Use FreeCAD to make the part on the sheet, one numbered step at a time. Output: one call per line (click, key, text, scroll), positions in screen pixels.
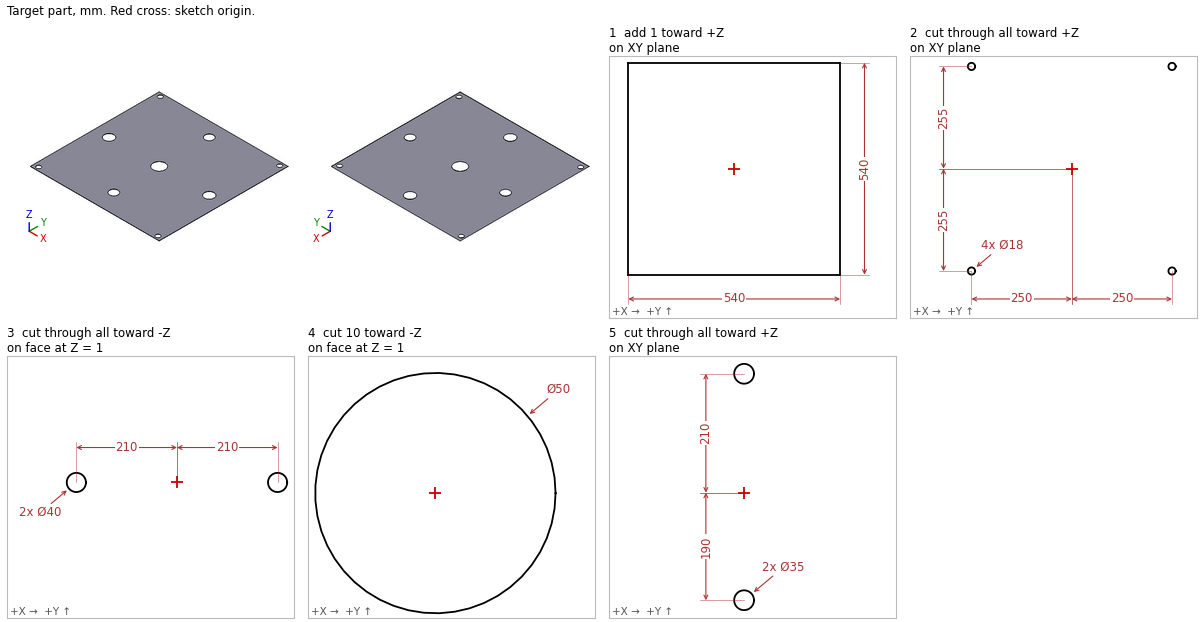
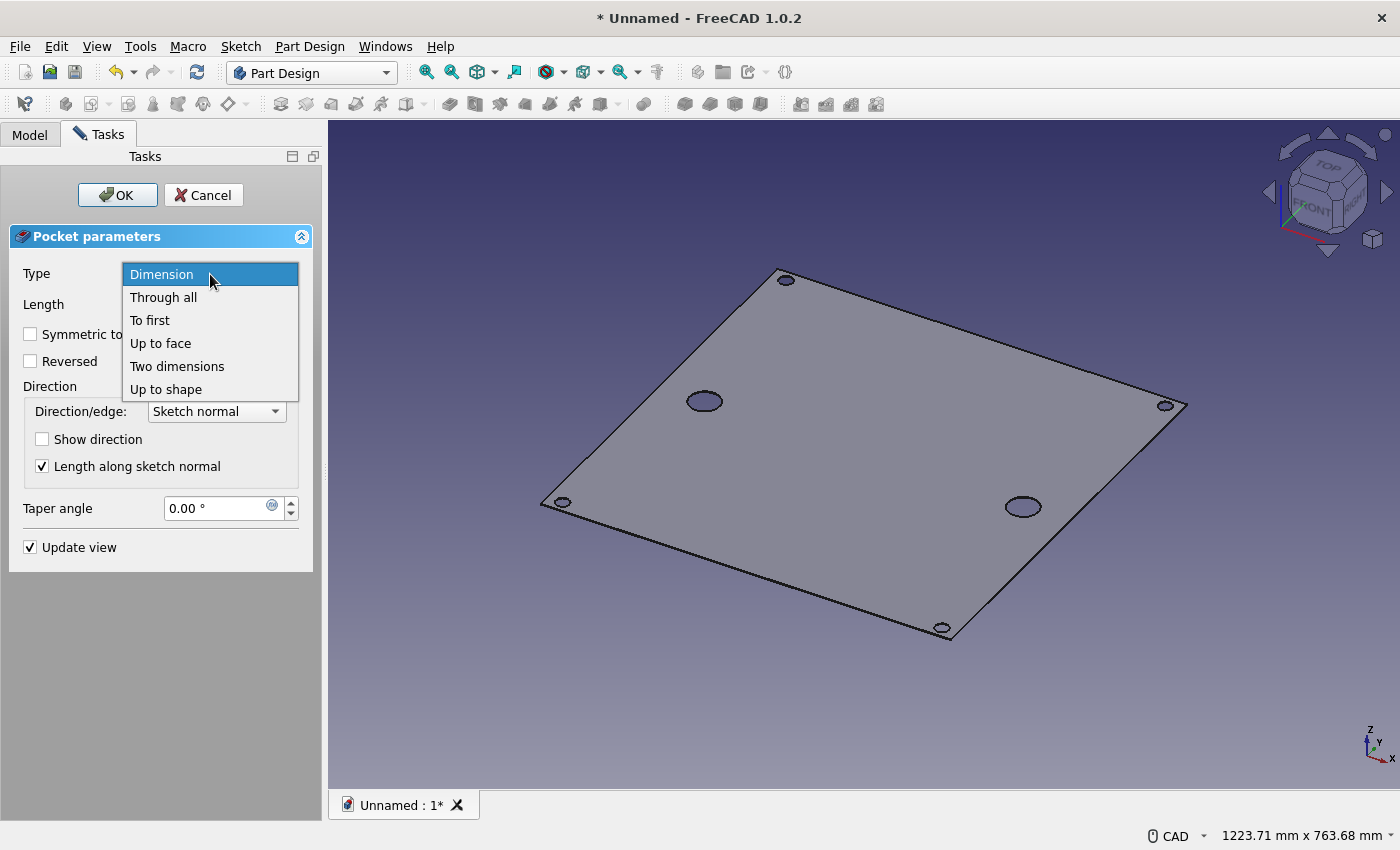
click(208, 298)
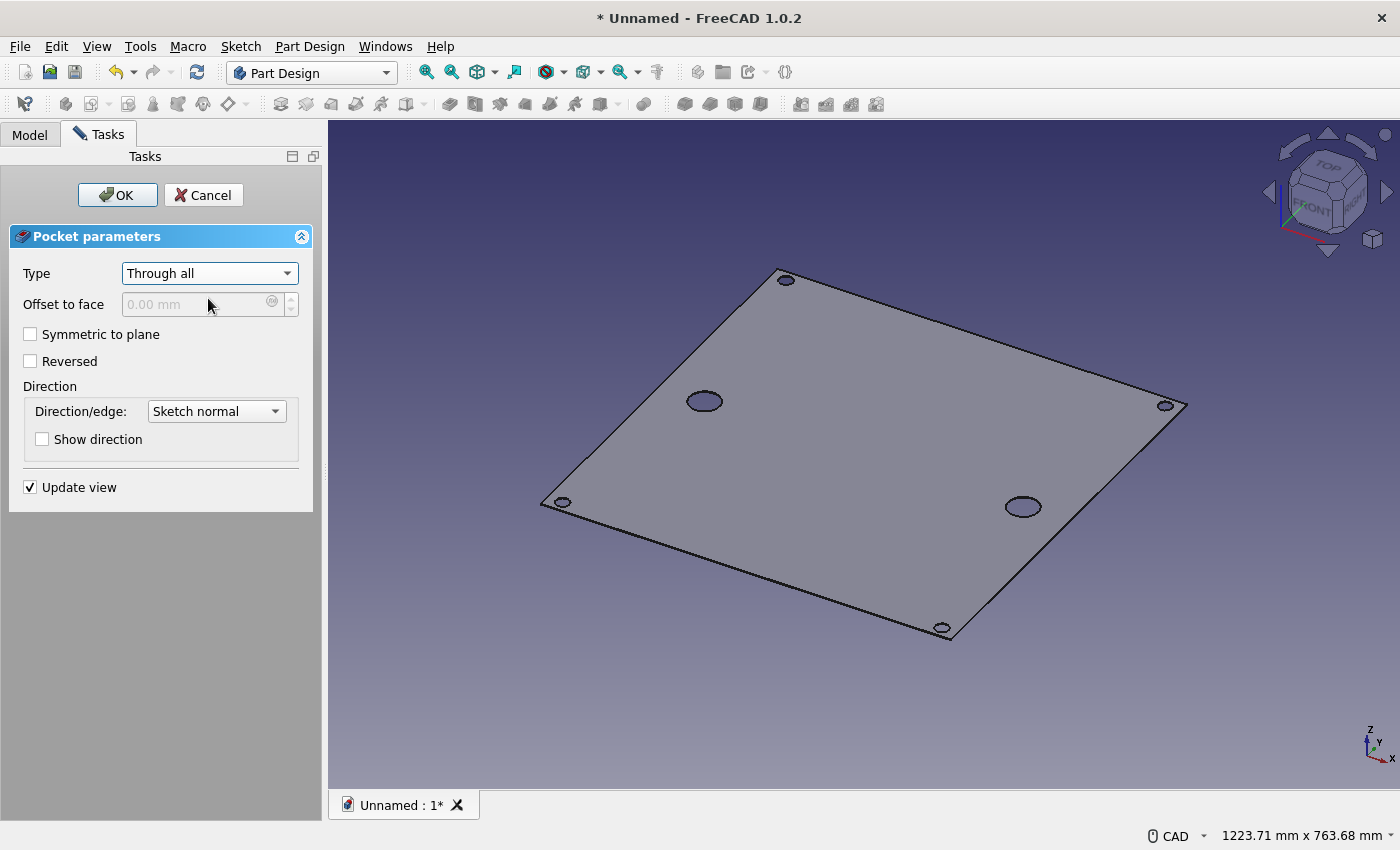
click(118, 195)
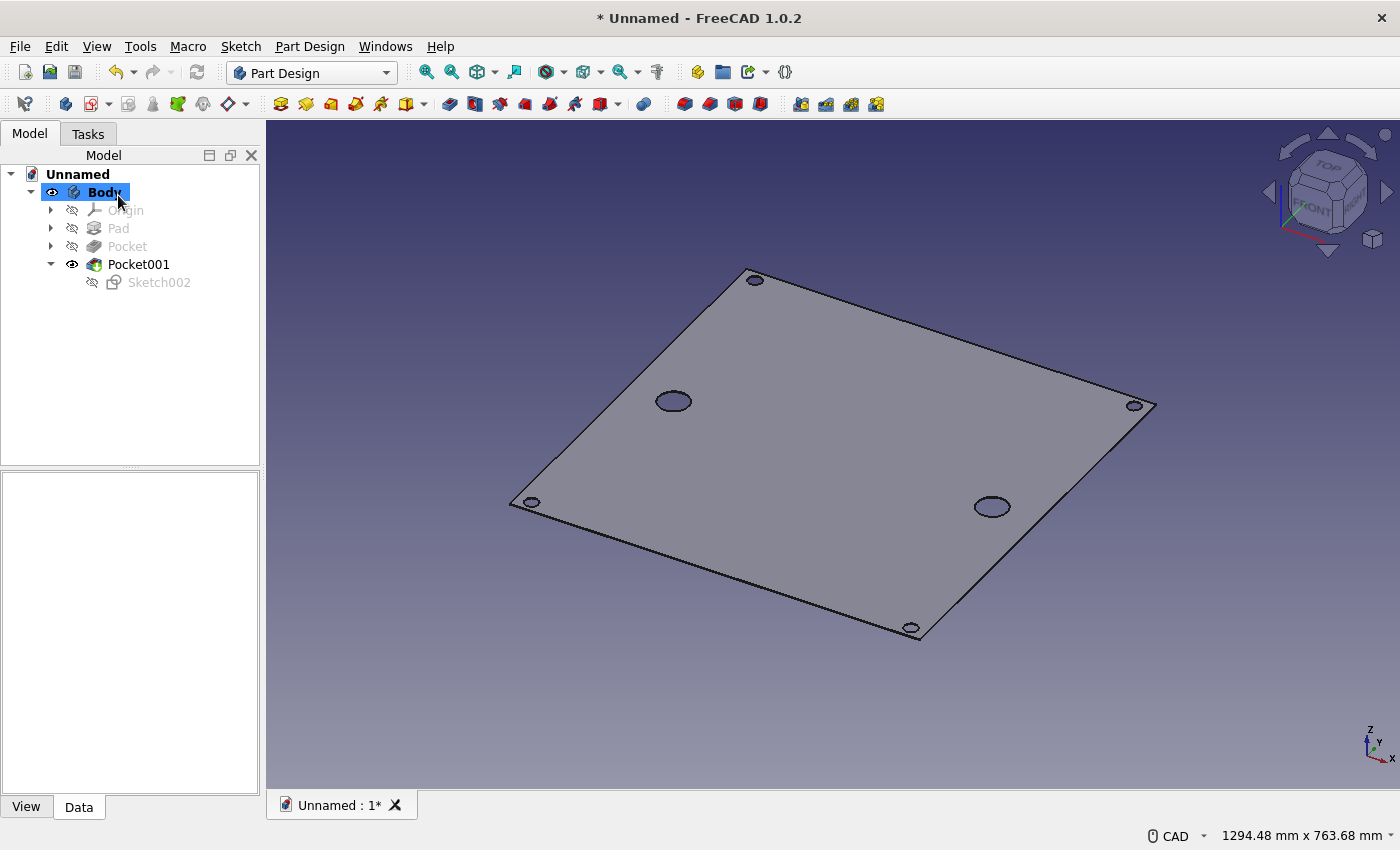
click(799, 487)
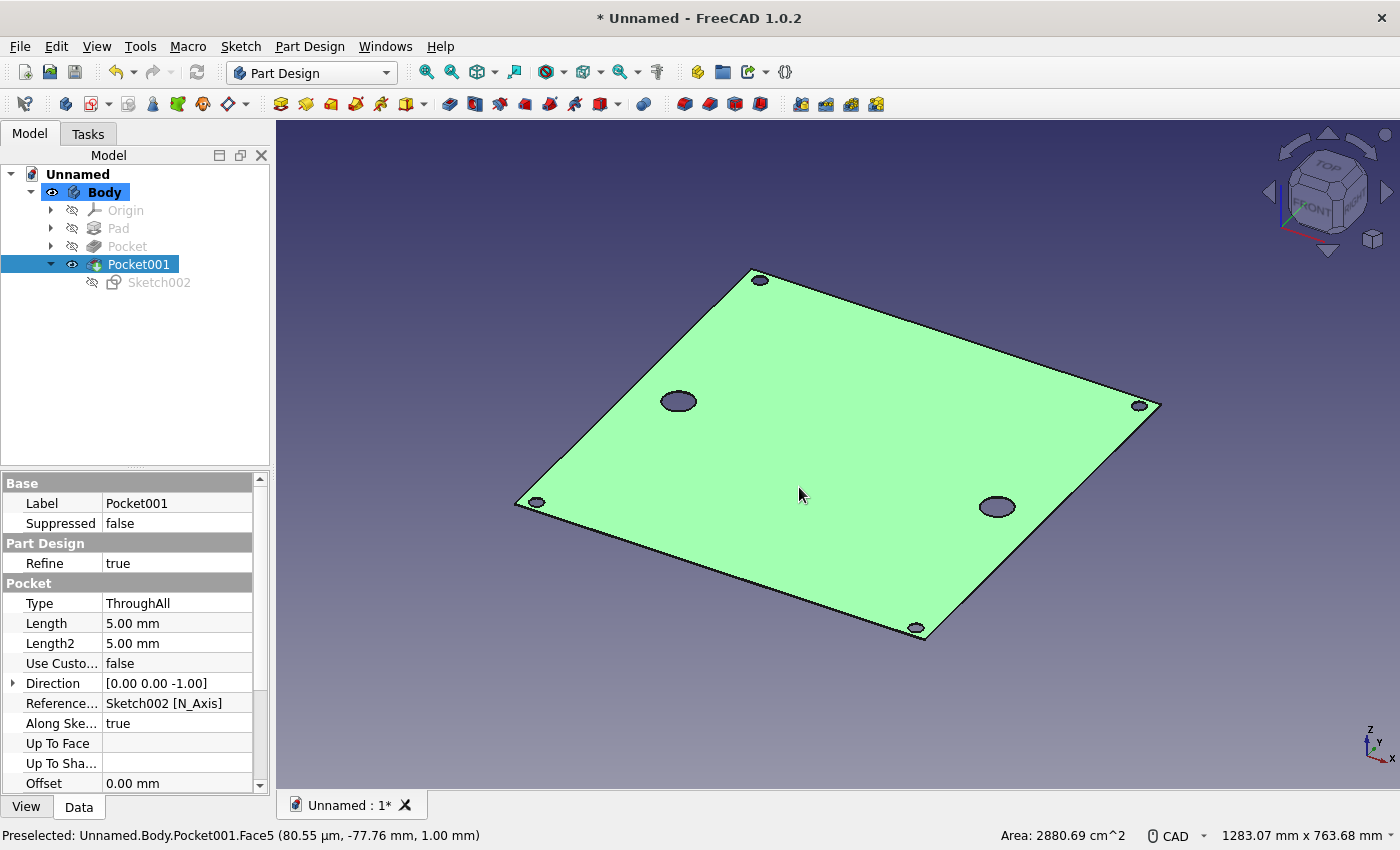
click(90, 104)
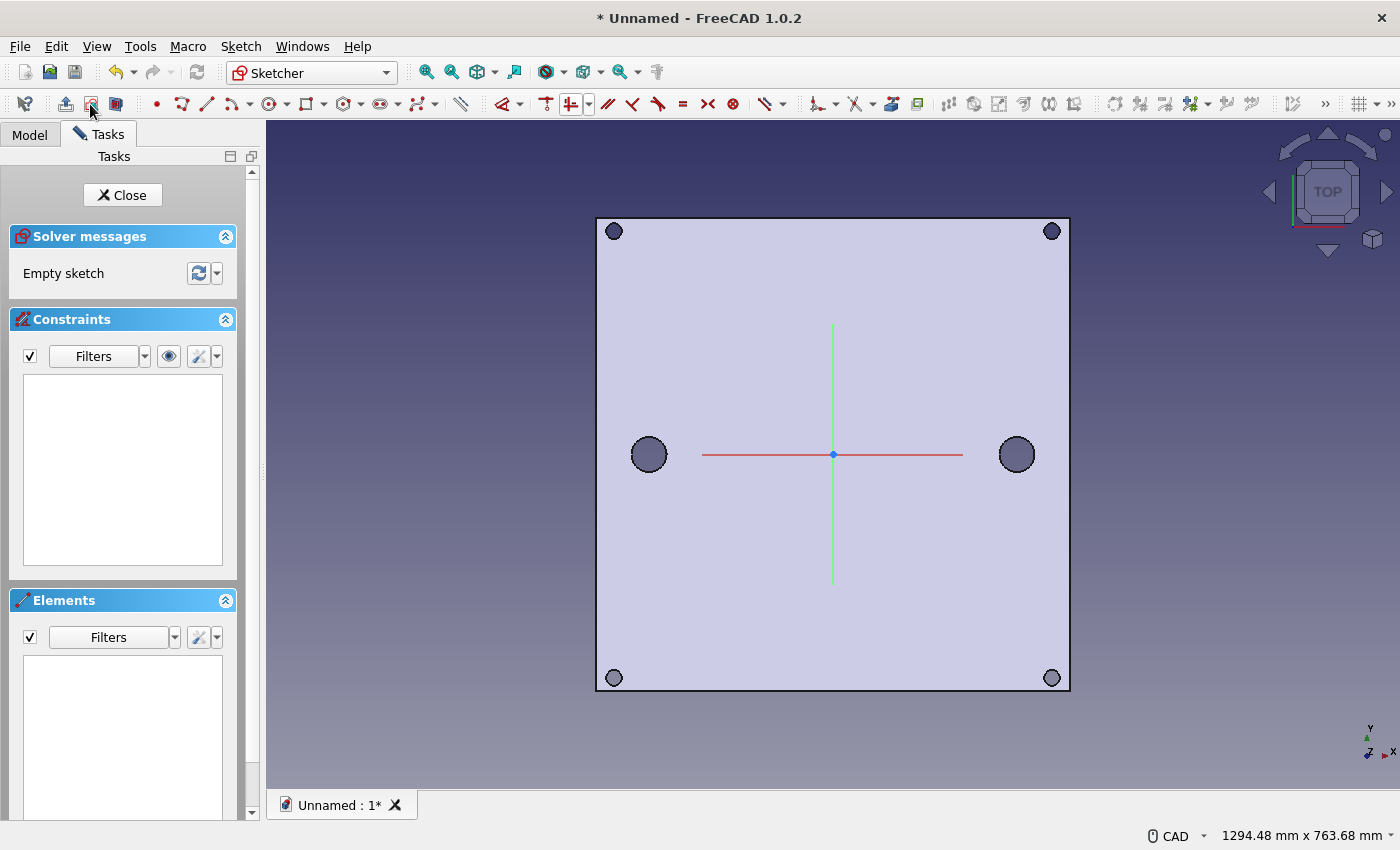
scroll(842, 454, up, 11)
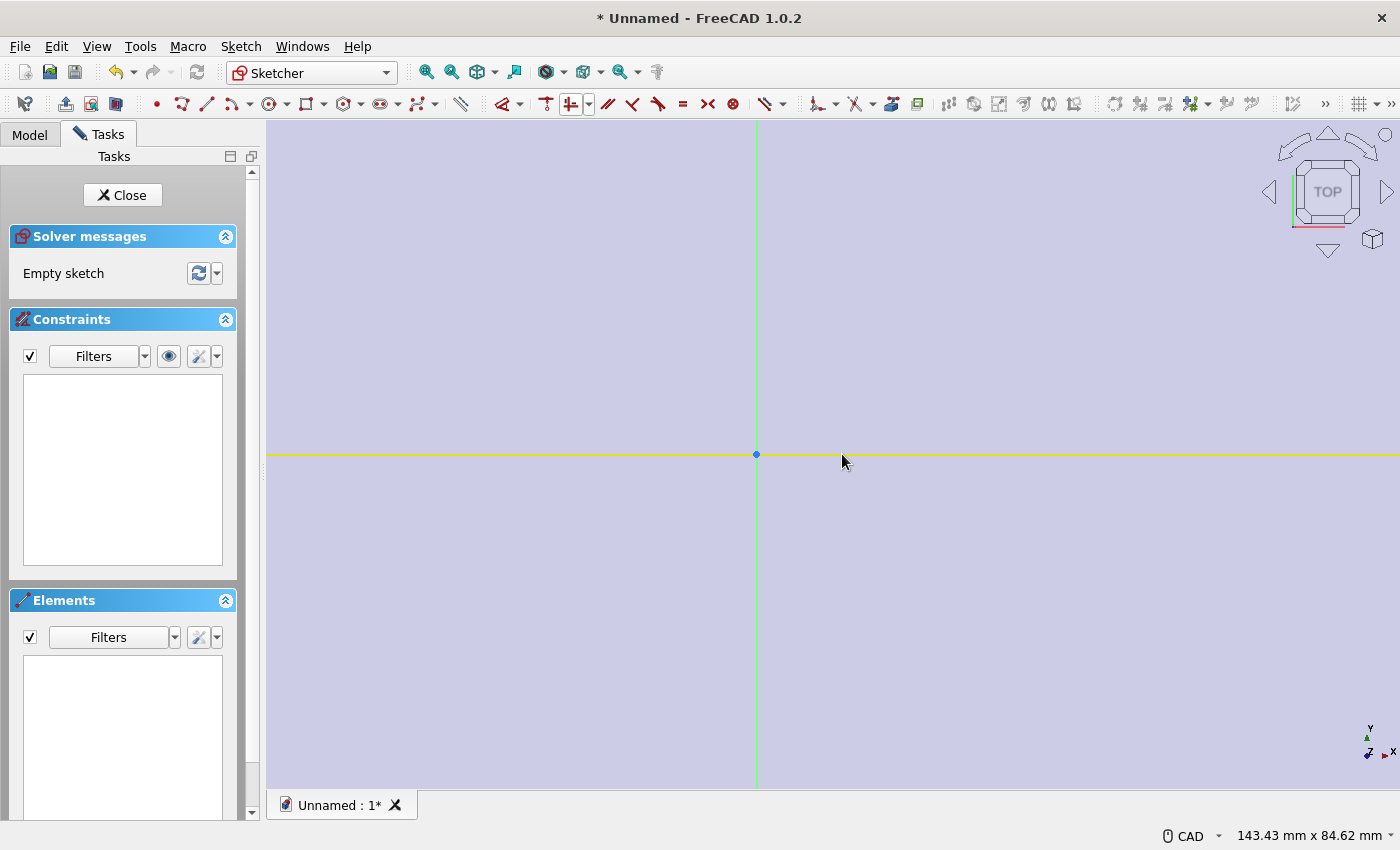
click(268, 104)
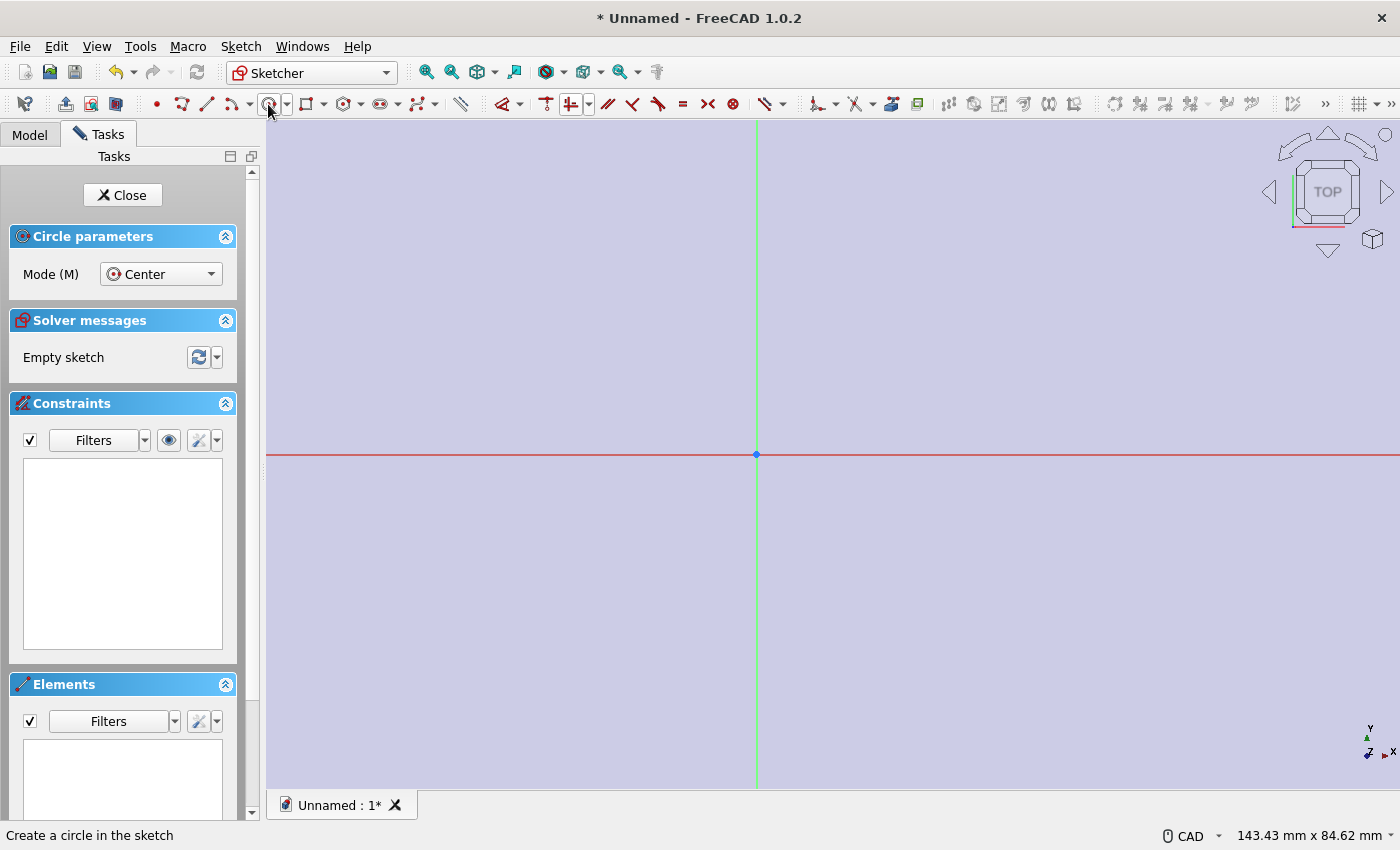
click(757, 454)
move(896, 315)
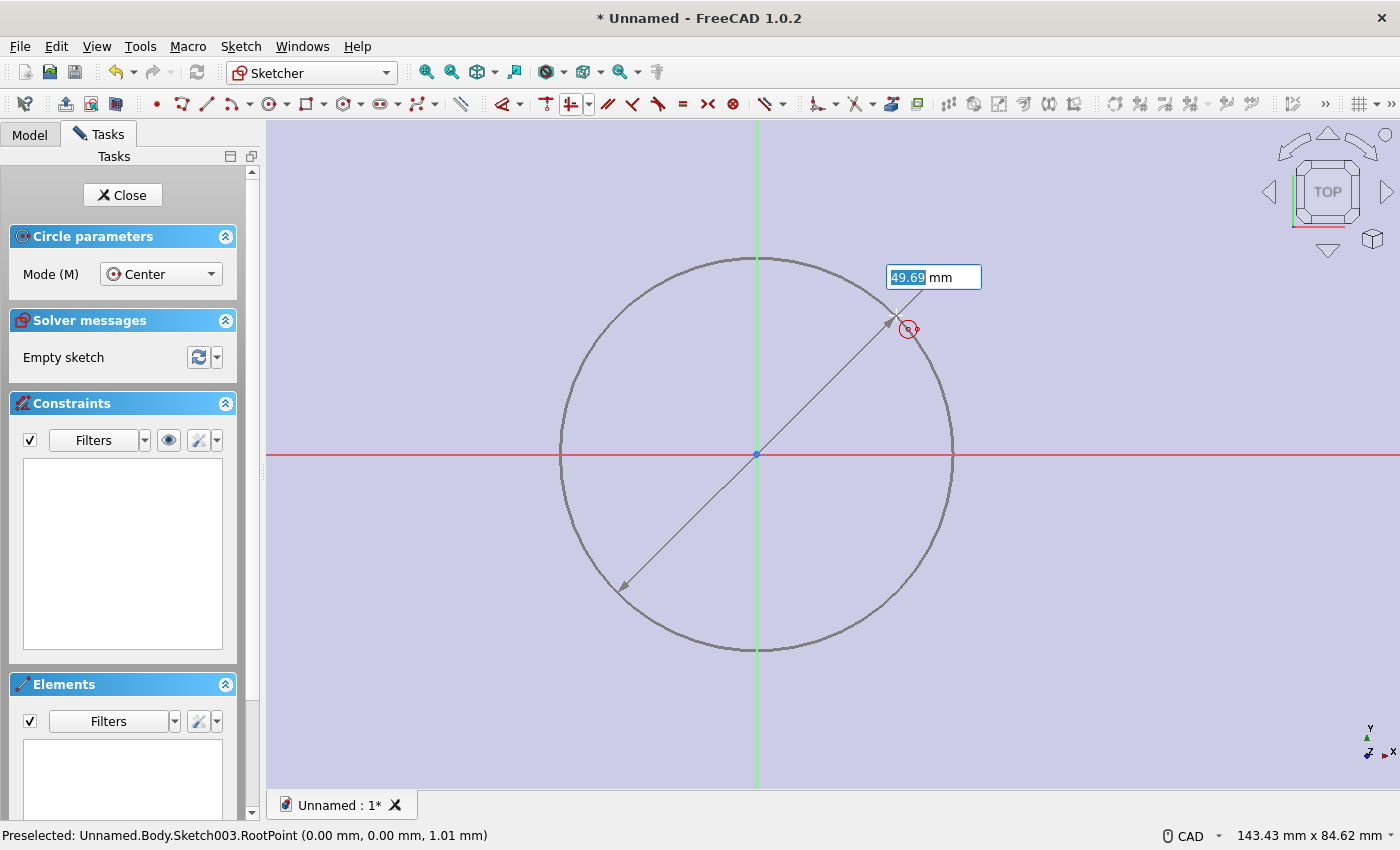
text(50)
key(Return)
key(Escape)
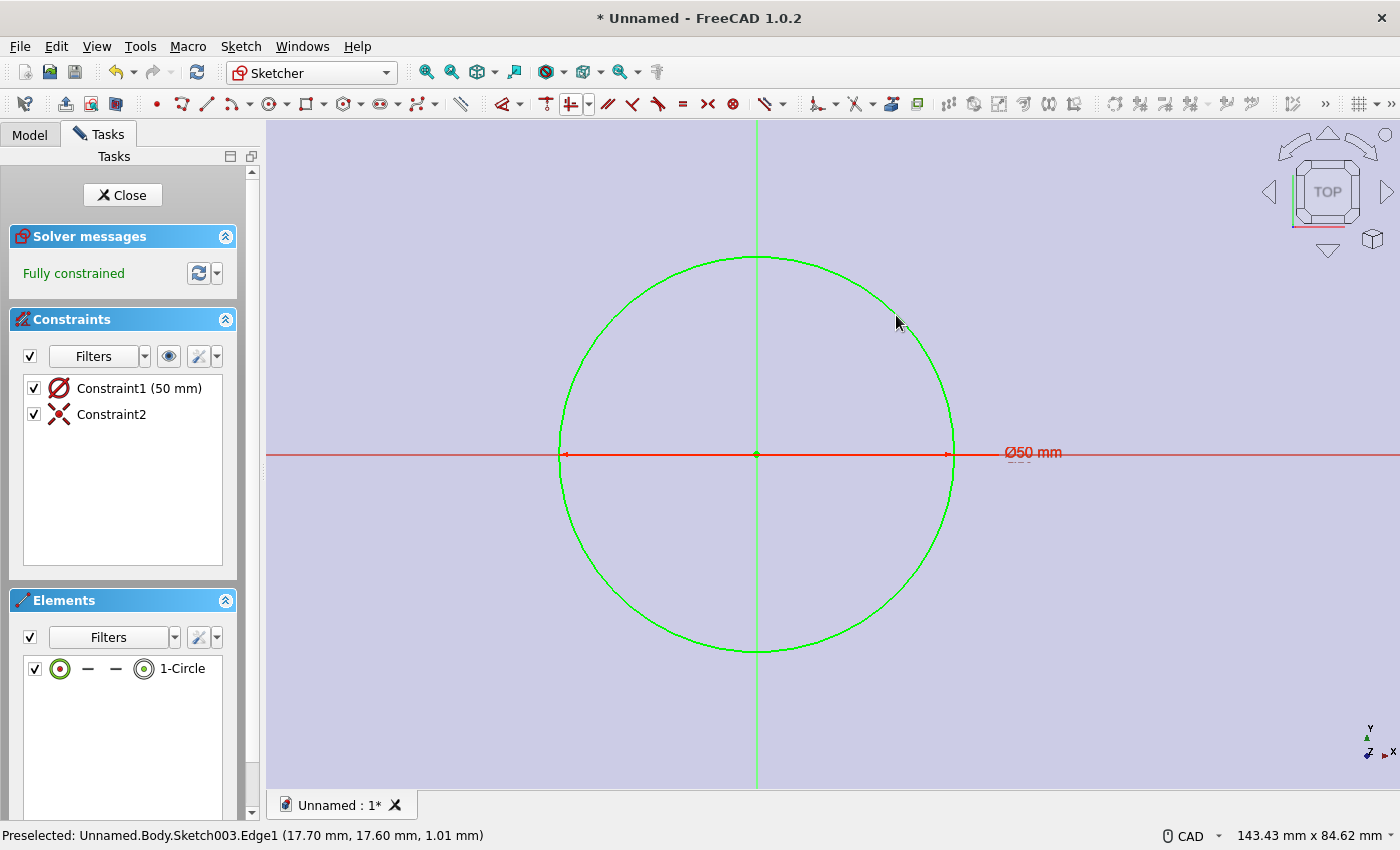
click(123, 195)